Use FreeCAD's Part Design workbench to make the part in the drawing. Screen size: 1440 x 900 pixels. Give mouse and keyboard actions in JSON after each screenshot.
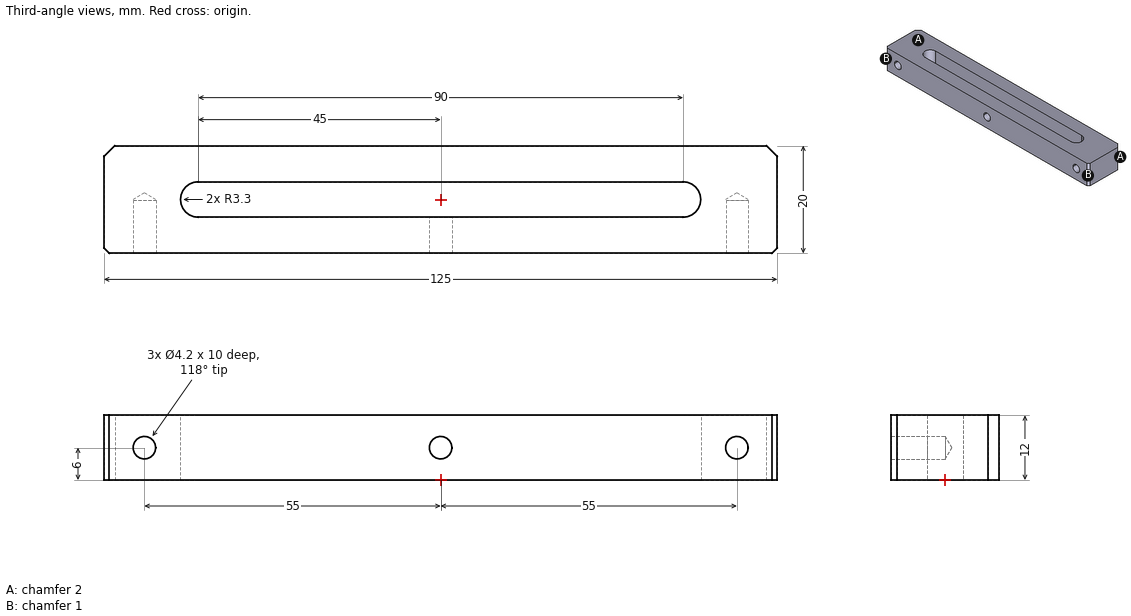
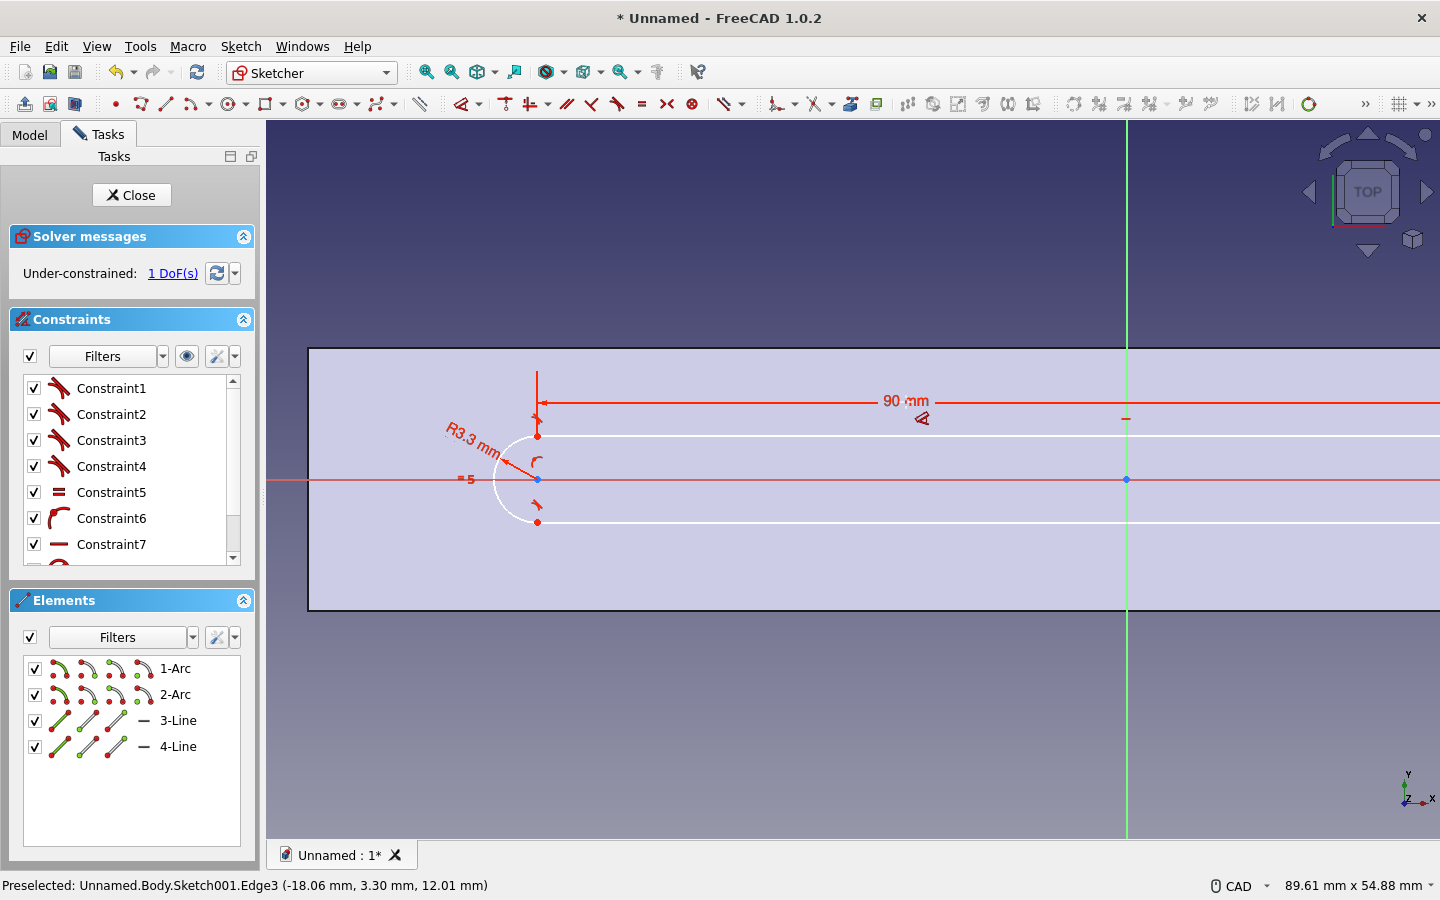
{"action": "left_click", "coordinate": [537, 436]}
{"action": "left_click", "coordinate": [832, 402]}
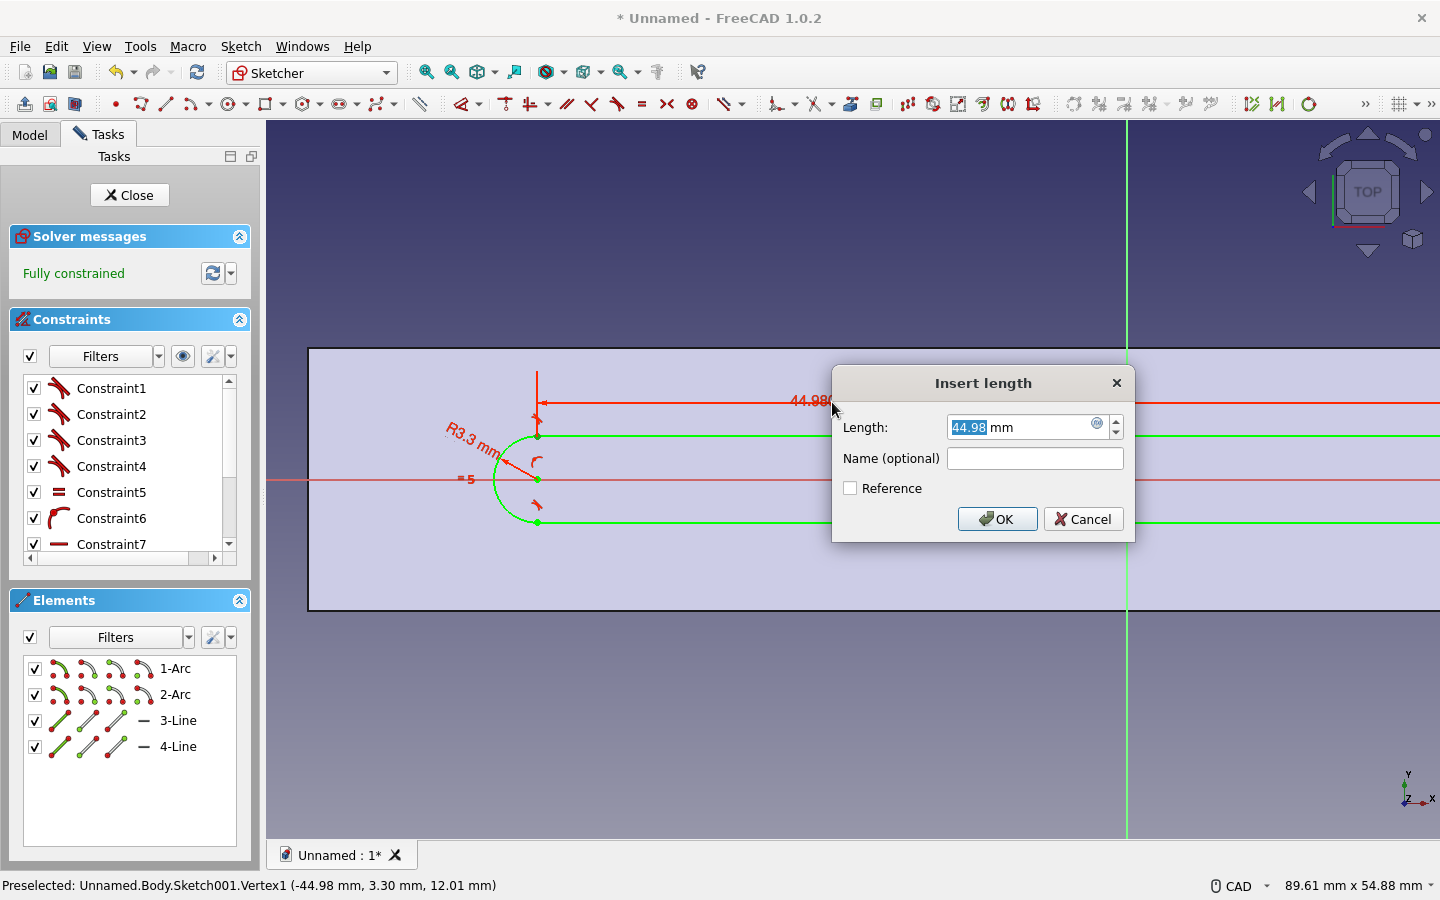
{"action": "type", "text": "45"}
{"action": "key", "text": "Return"}
{"action": "key", "text": "Escape"}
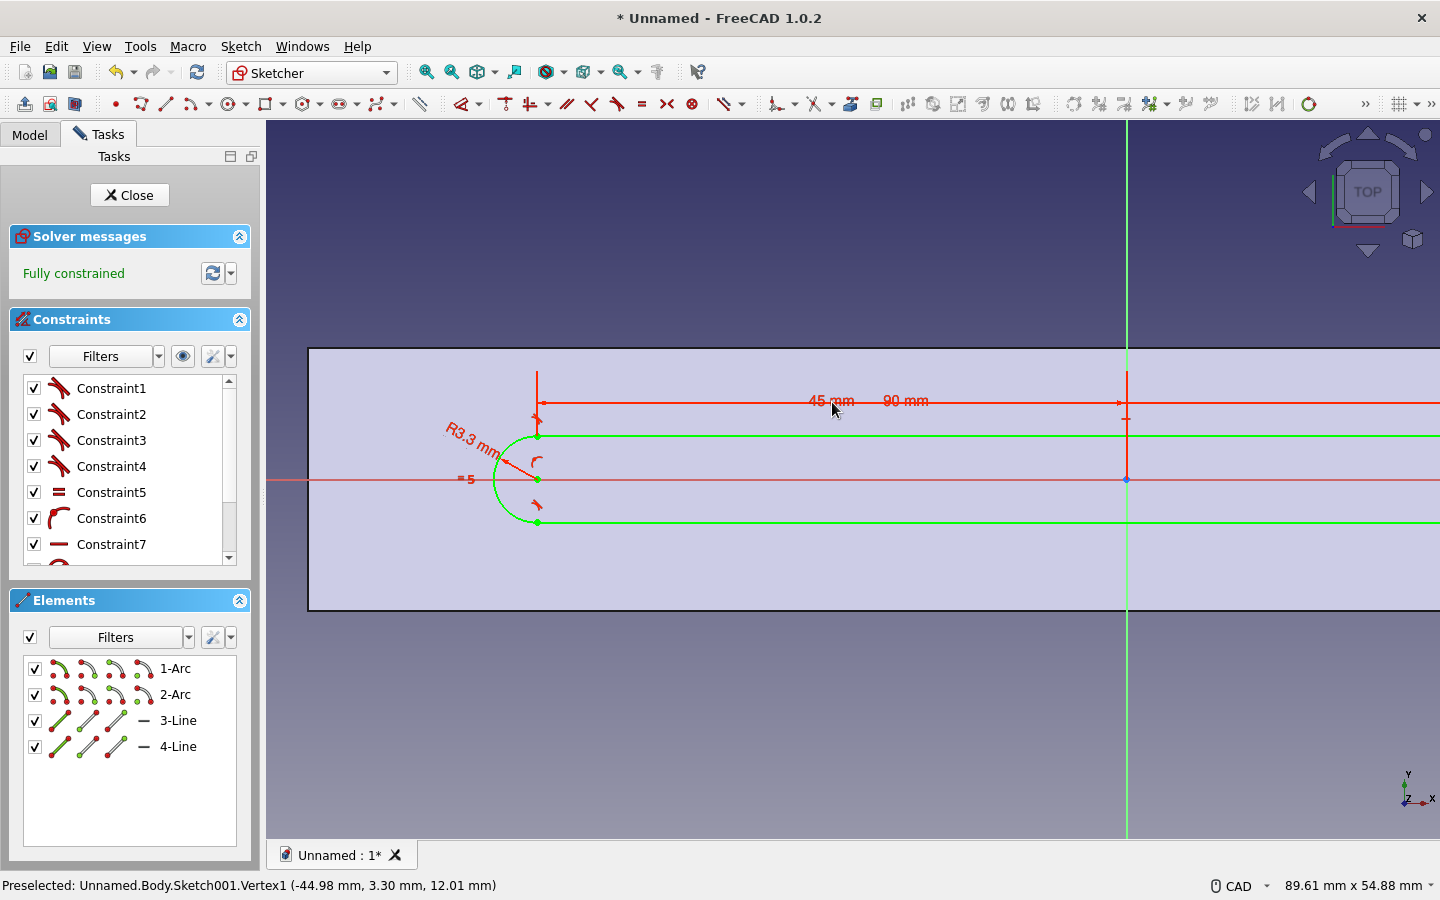
{"action": "left_click", "coordinate": [130, 195]}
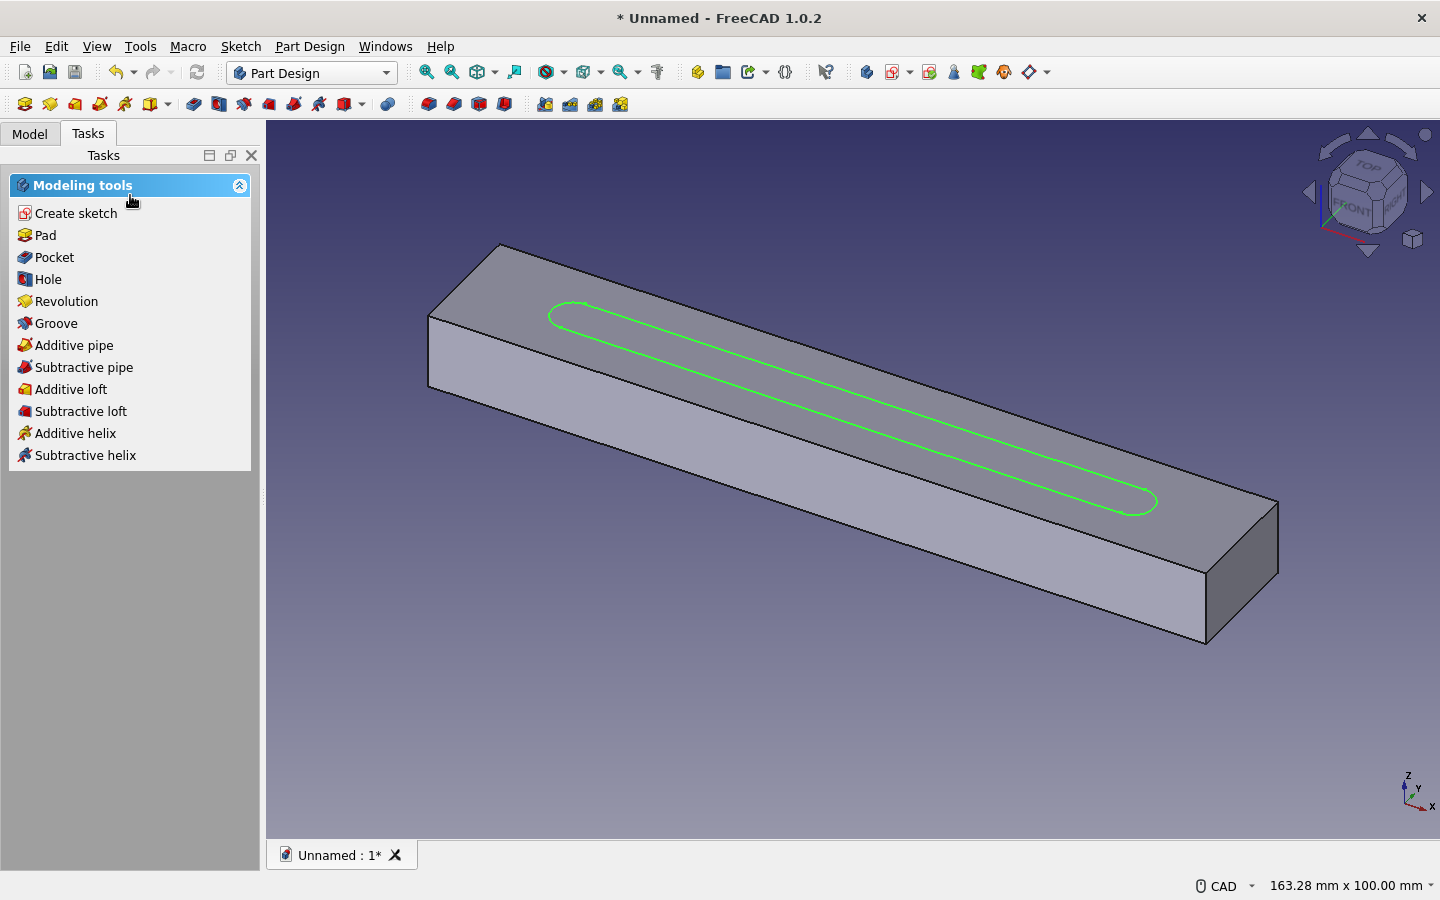
{"action": "left_click", "coordinate": [194, 104]}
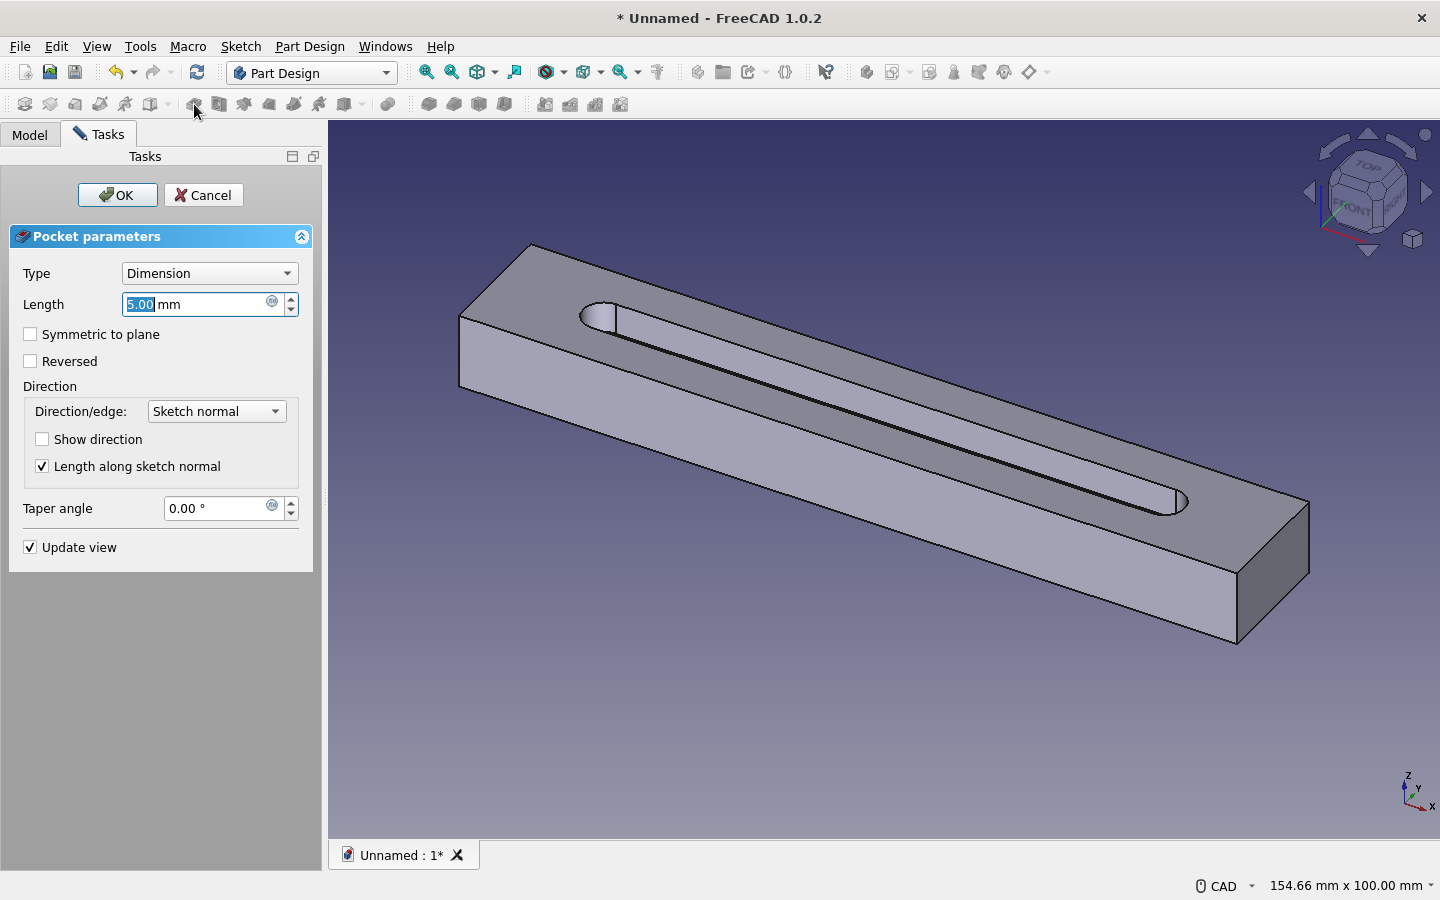
{"action": "left_click", "coordinate": [210, 274]}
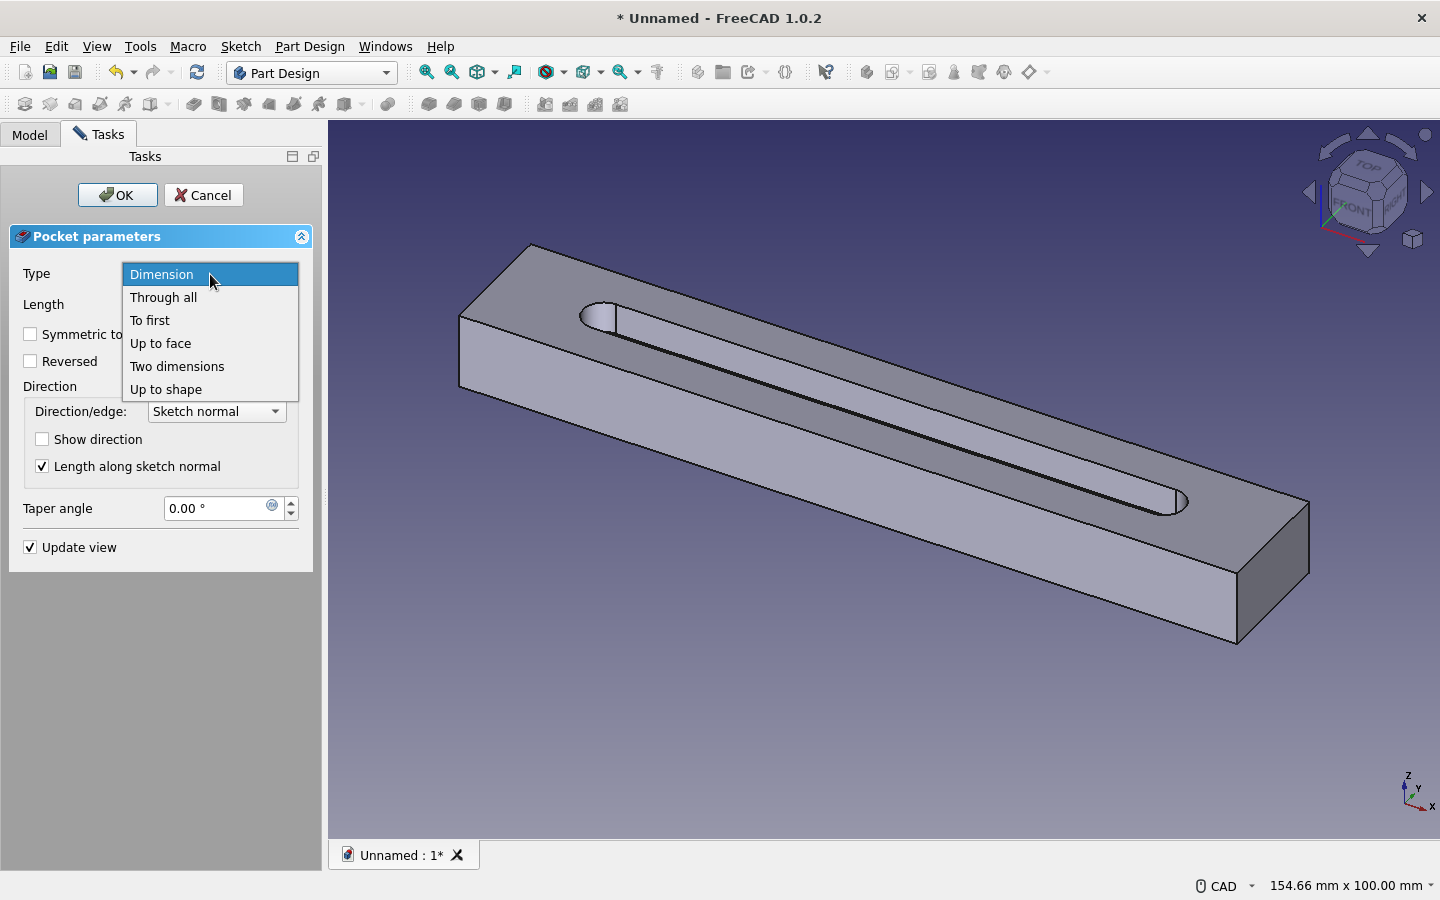
{"action": "left_click", "coordinate": [208, 298]}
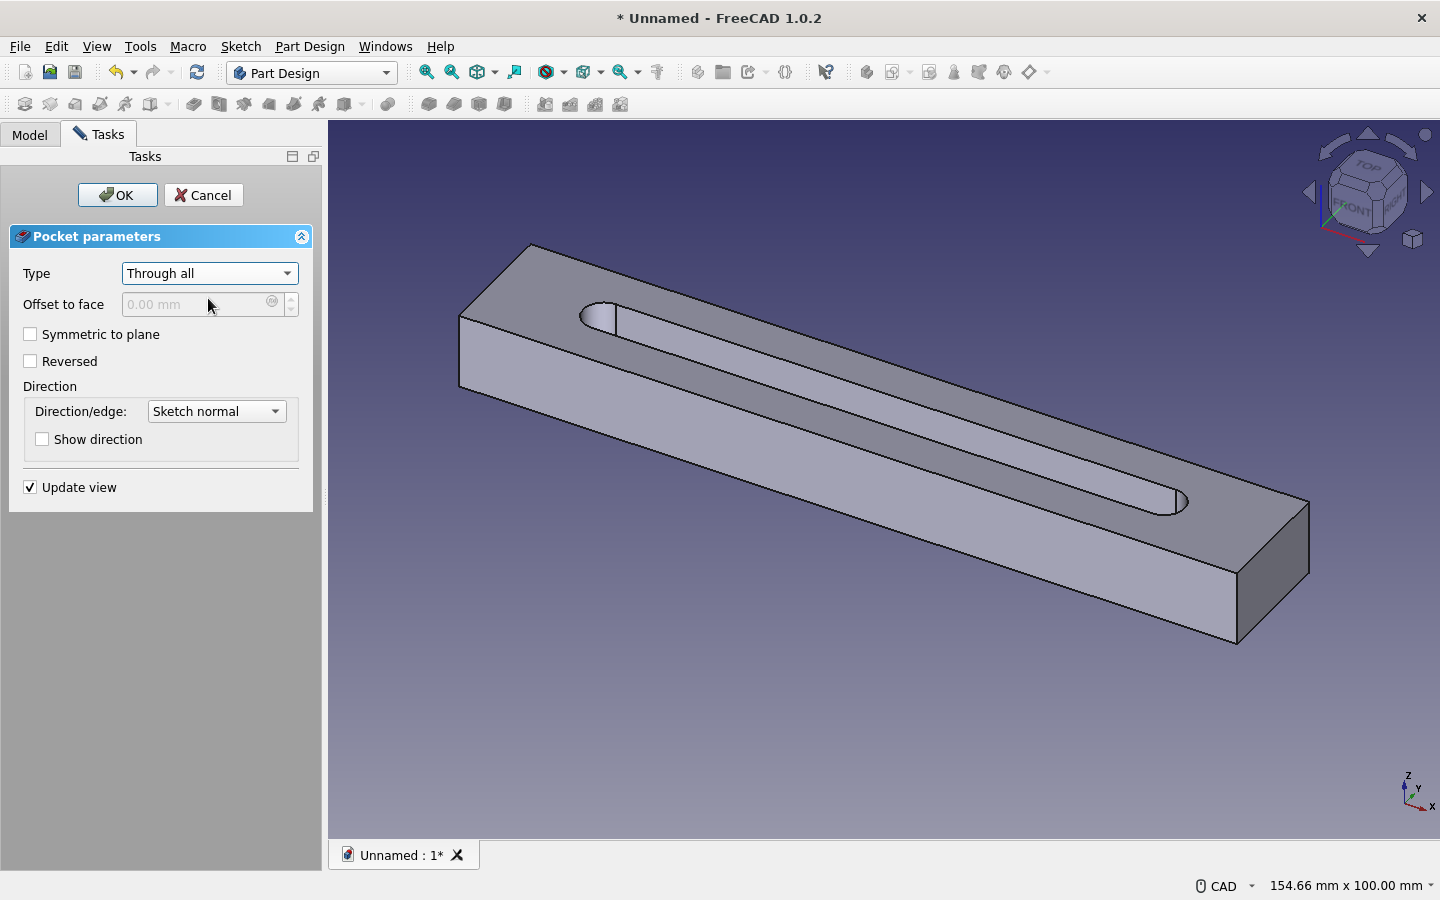
{"action": "left_click", "coordinate": [118, 195]}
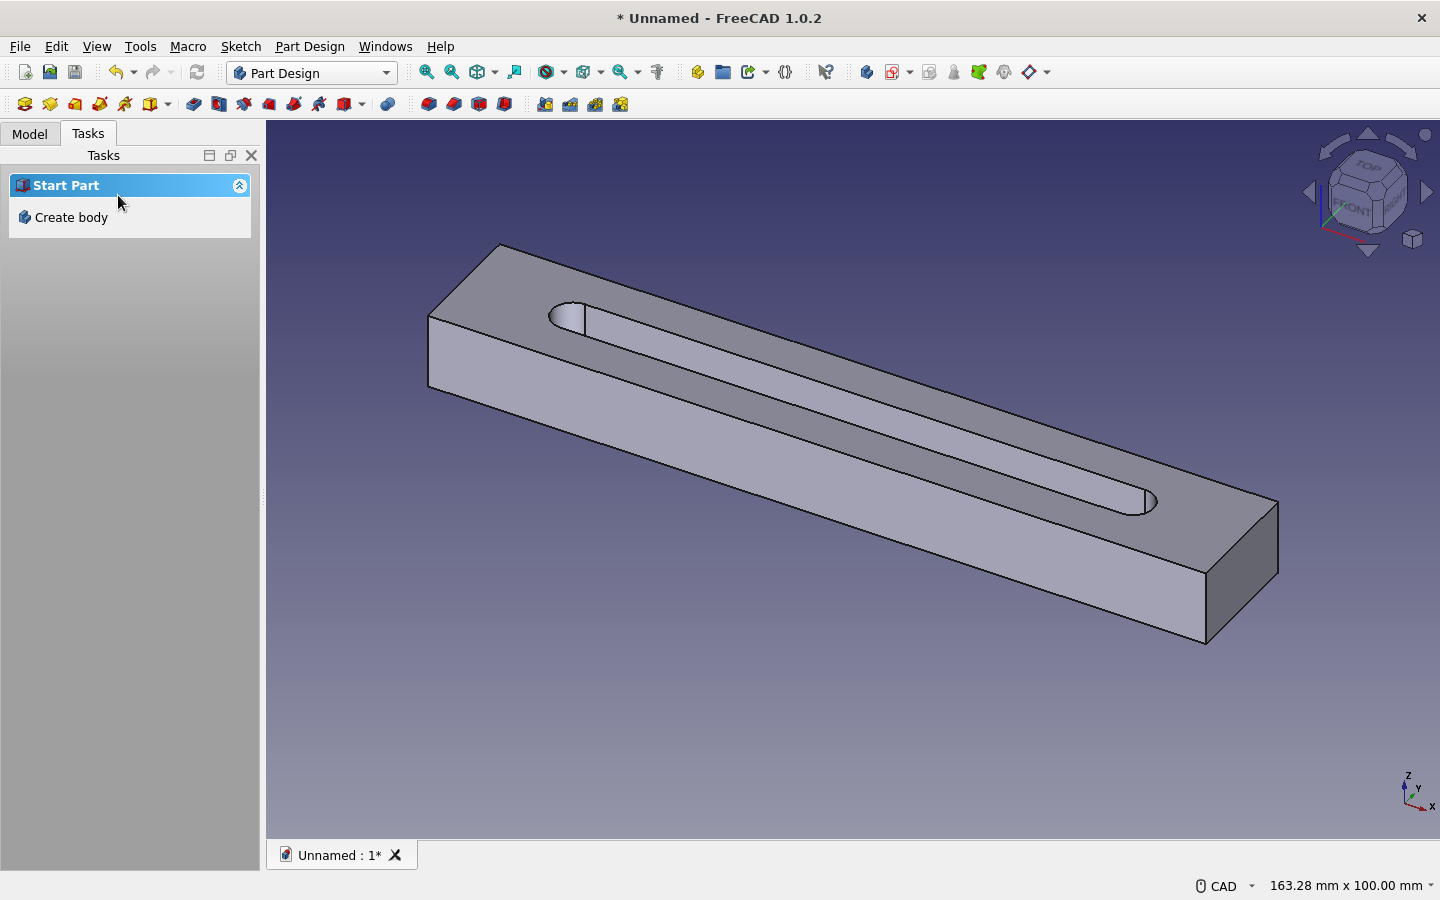
{"action": "left_click", "coordinate": [1151, 589]}